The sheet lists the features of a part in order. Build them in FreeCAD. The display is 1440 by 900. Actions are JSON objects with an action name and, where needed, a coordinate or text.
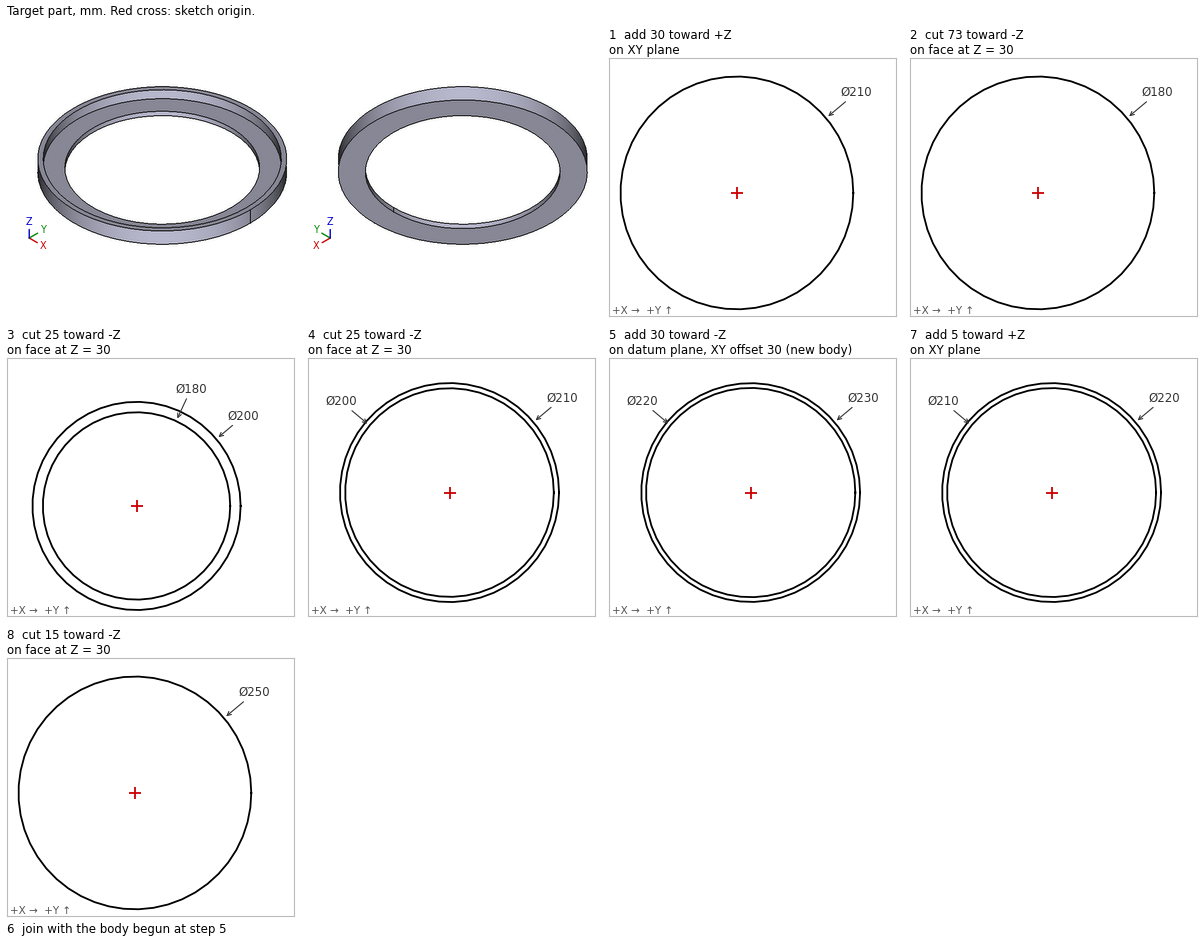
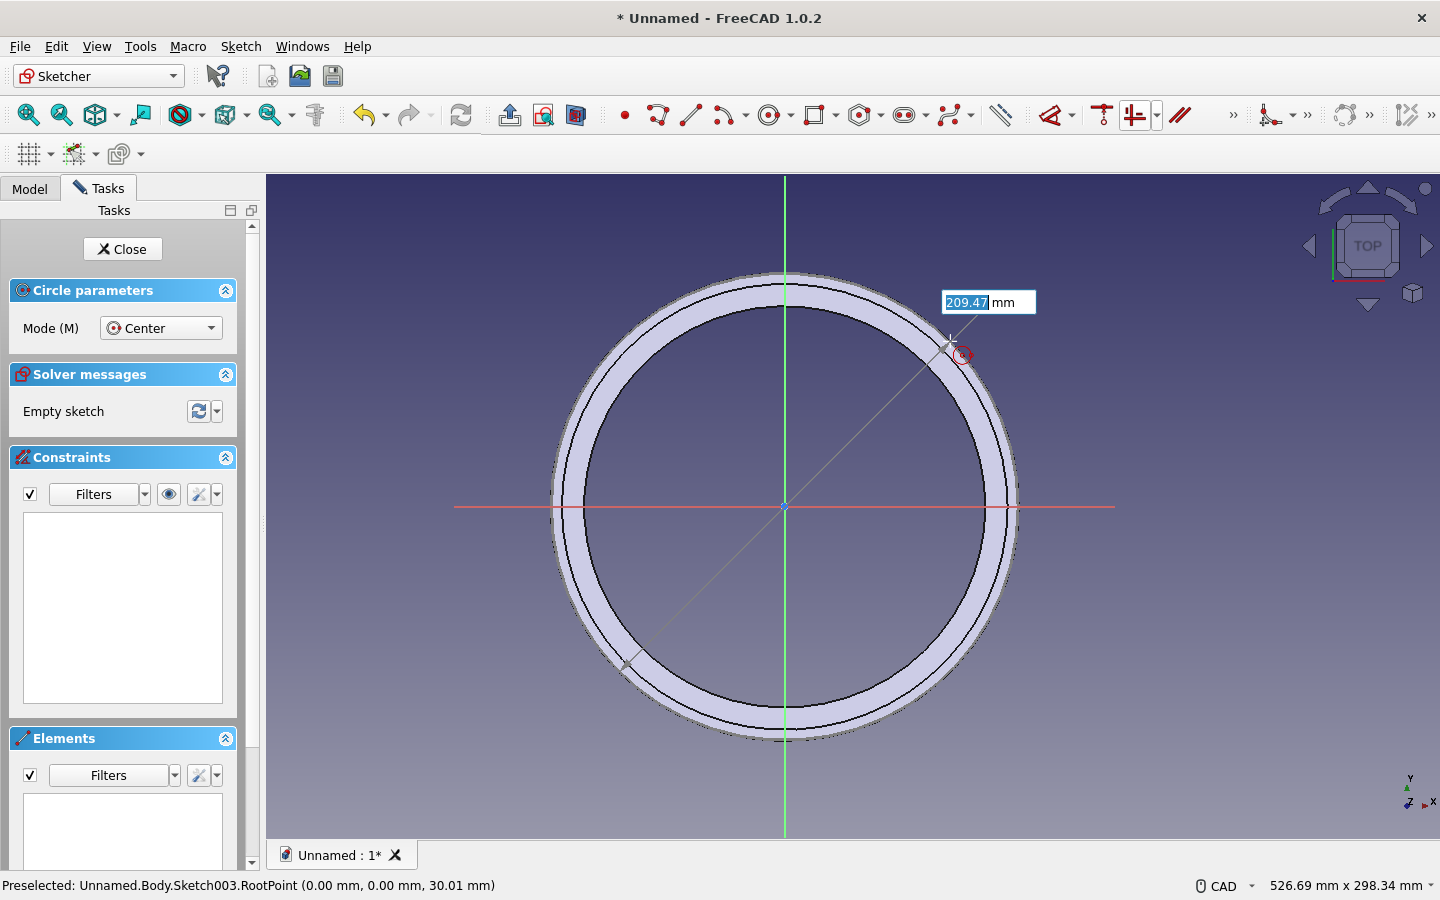
{"action": "type", "text": "210"}
{"action": "key", "text": "Return"}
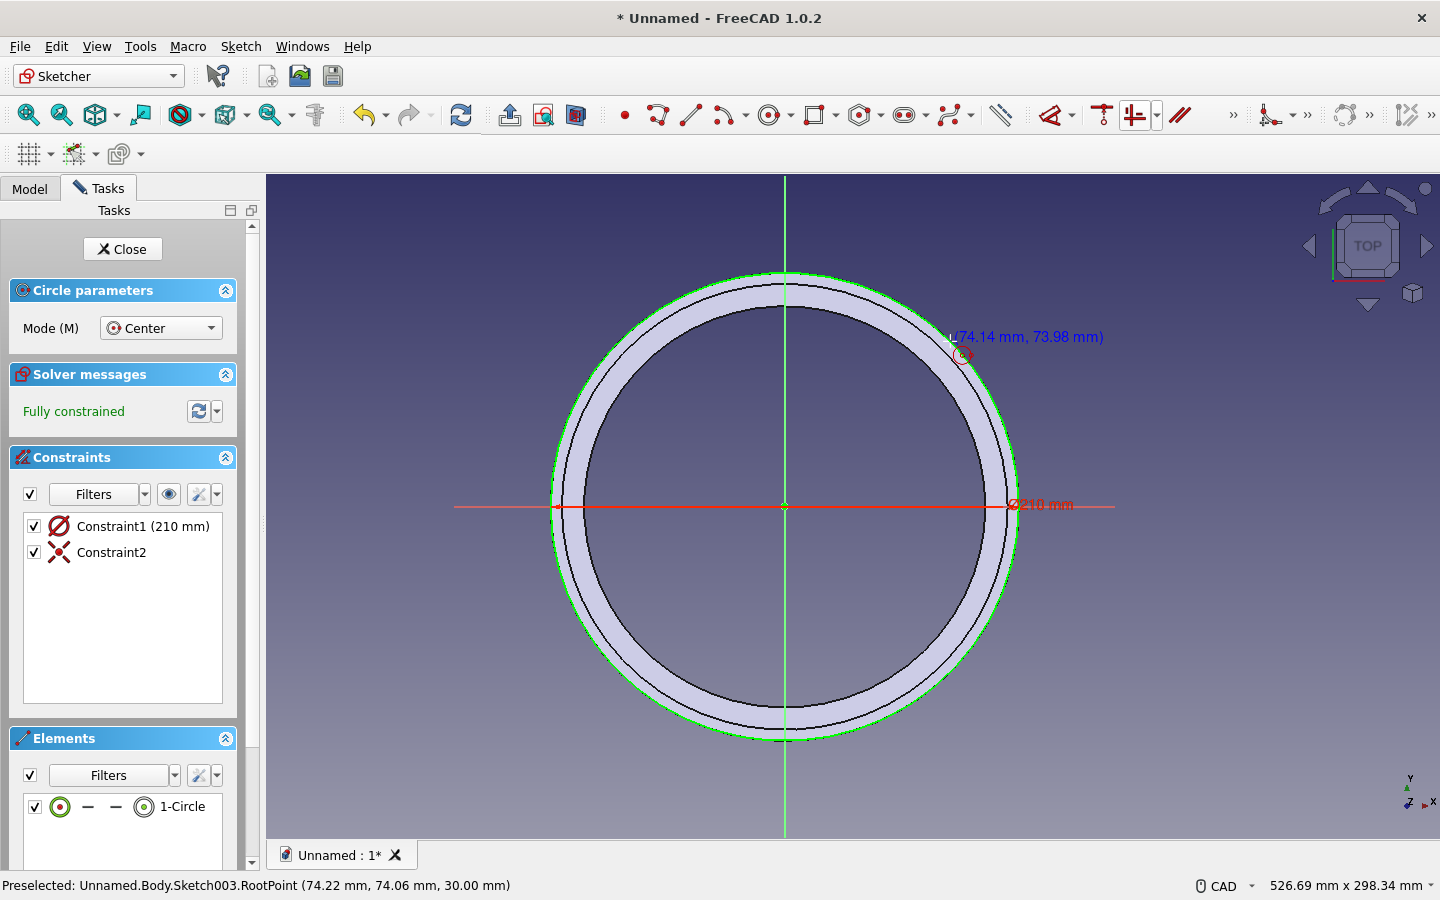
{"action": "left_click", "coordinate": [785, 507]}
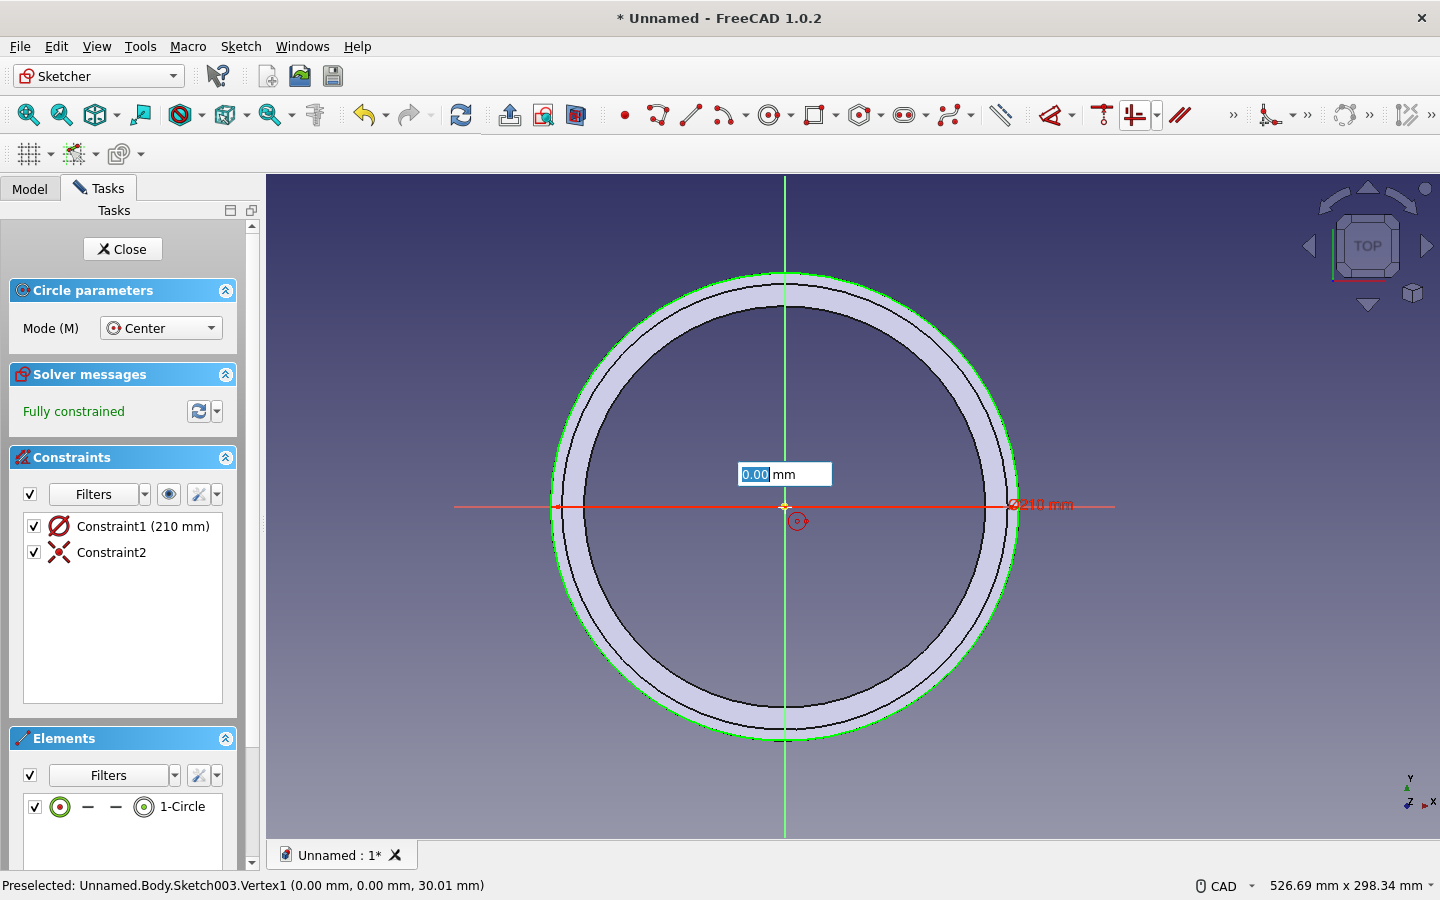
{"action": "scroll", "coordinate": [942, 349], "scroll_direction": "up", "scroll_amount": 2}
{"action": "mouse_move", "coordinate": [942, 349]}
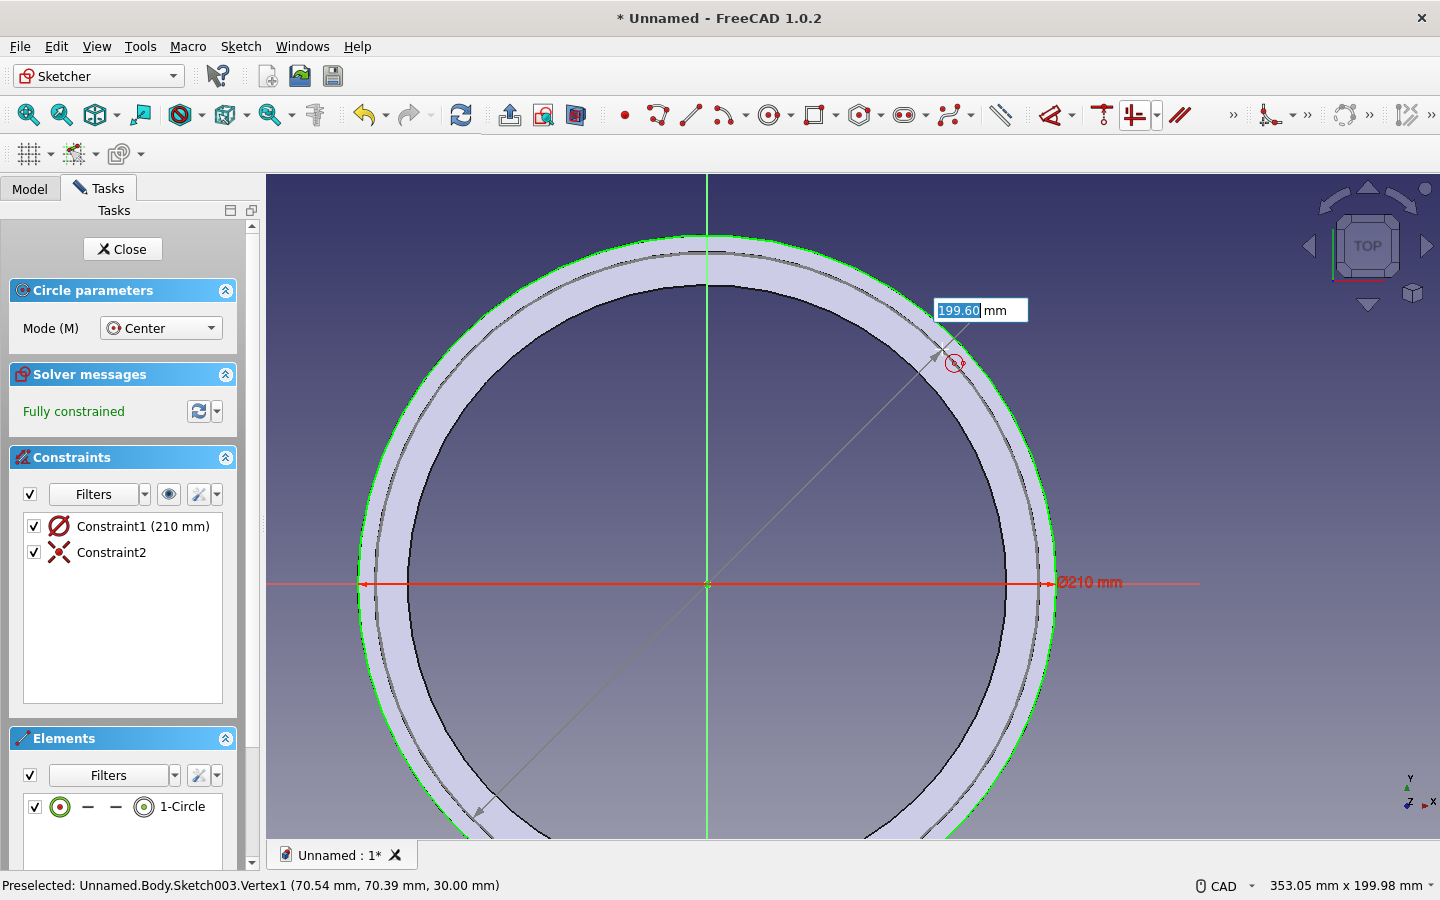
{"action": "type", "text": "200"}
{"action": "key", "text": "Return"}
{"action": "key", "text": "Escape"}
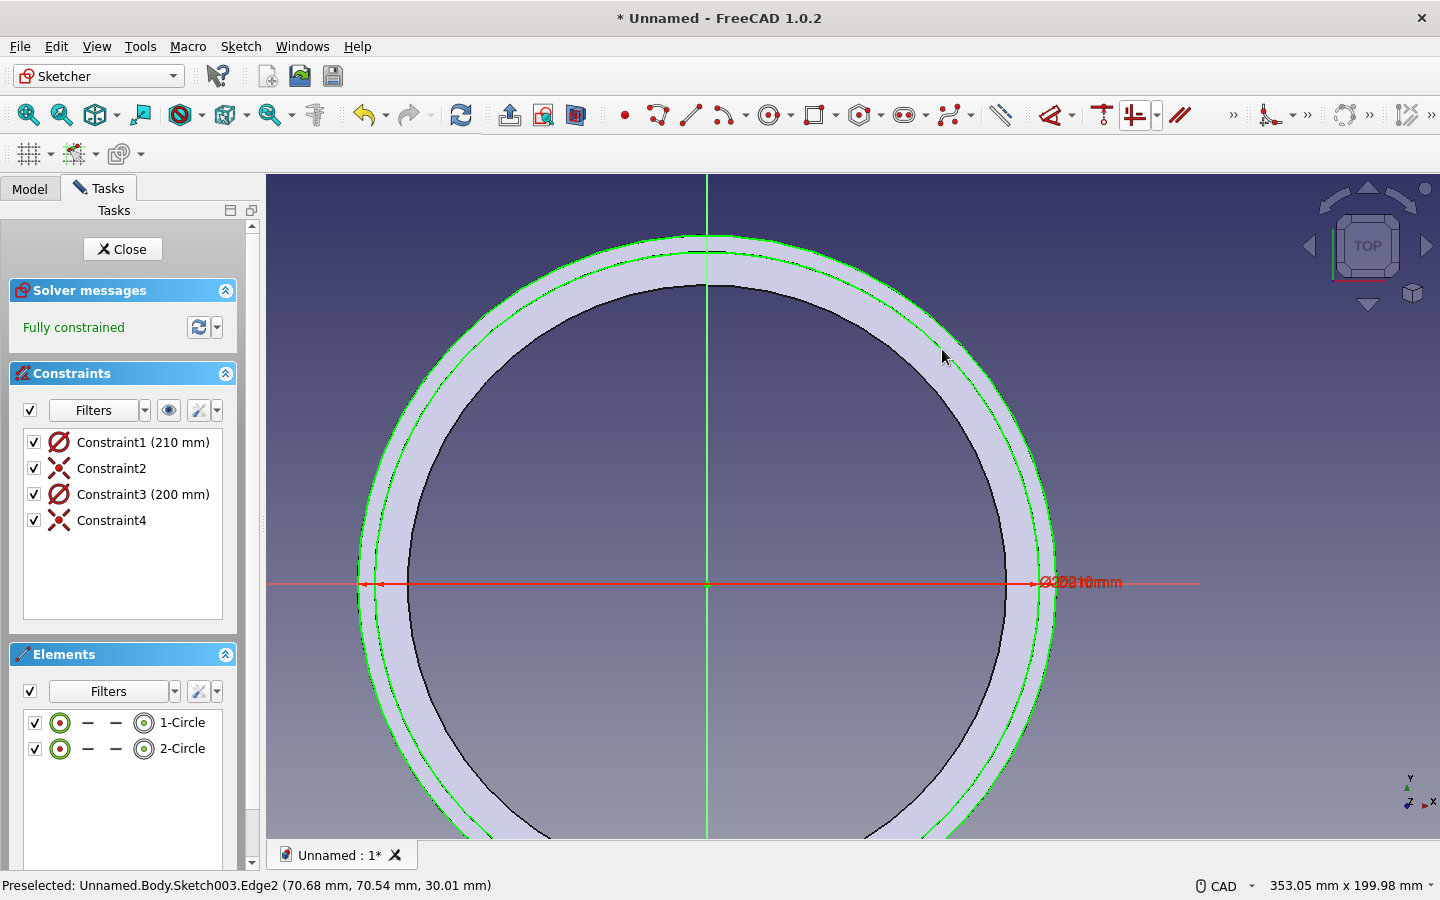
{"action": "left_click", "coordinate": [123, 249]}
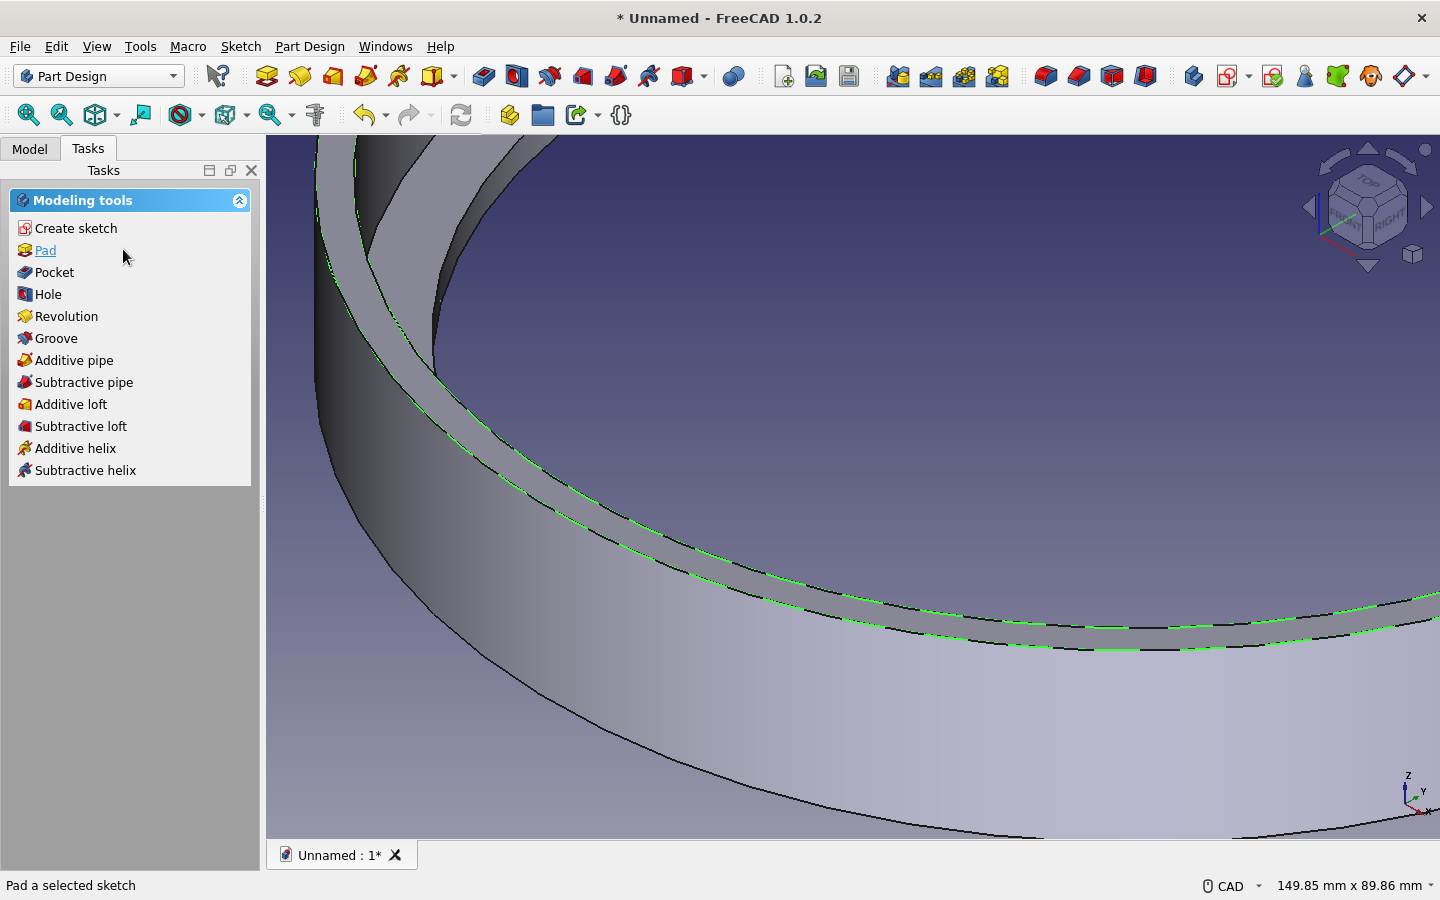
{"action": "left_click", "coordinate": [484, 76]}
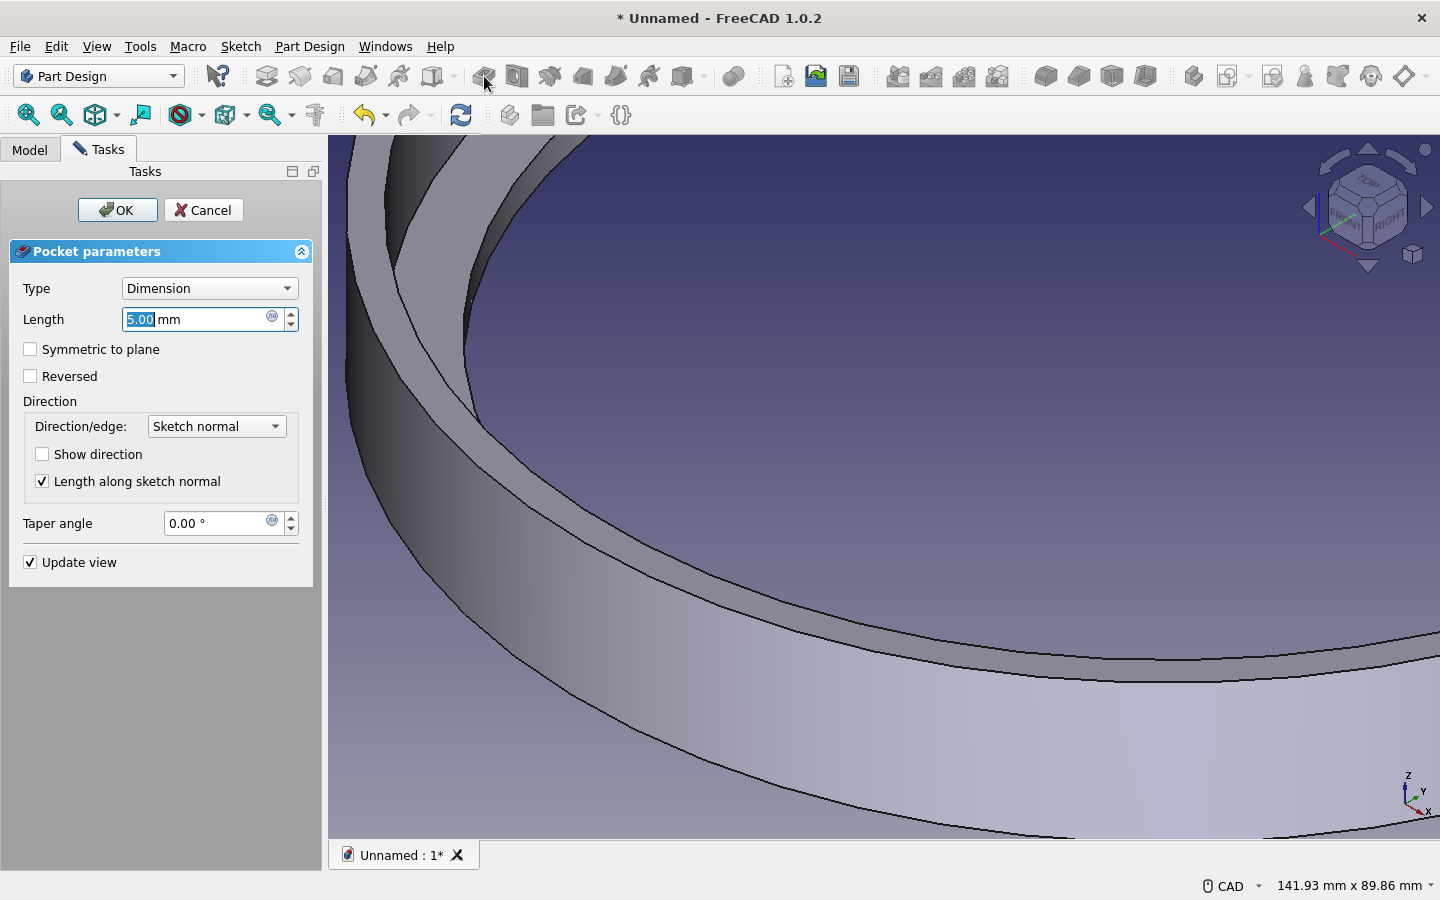
{"action": "type", "text": "25"}
{"action": "key", "text": "Tab"}